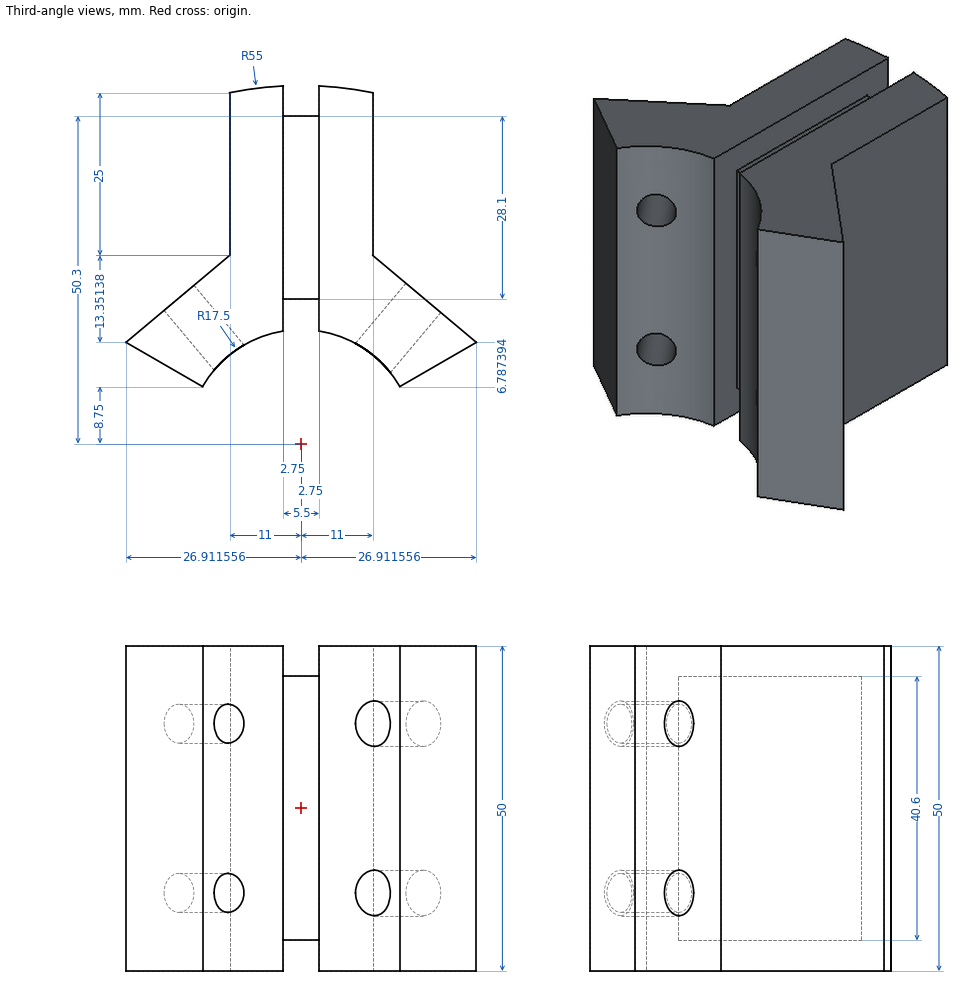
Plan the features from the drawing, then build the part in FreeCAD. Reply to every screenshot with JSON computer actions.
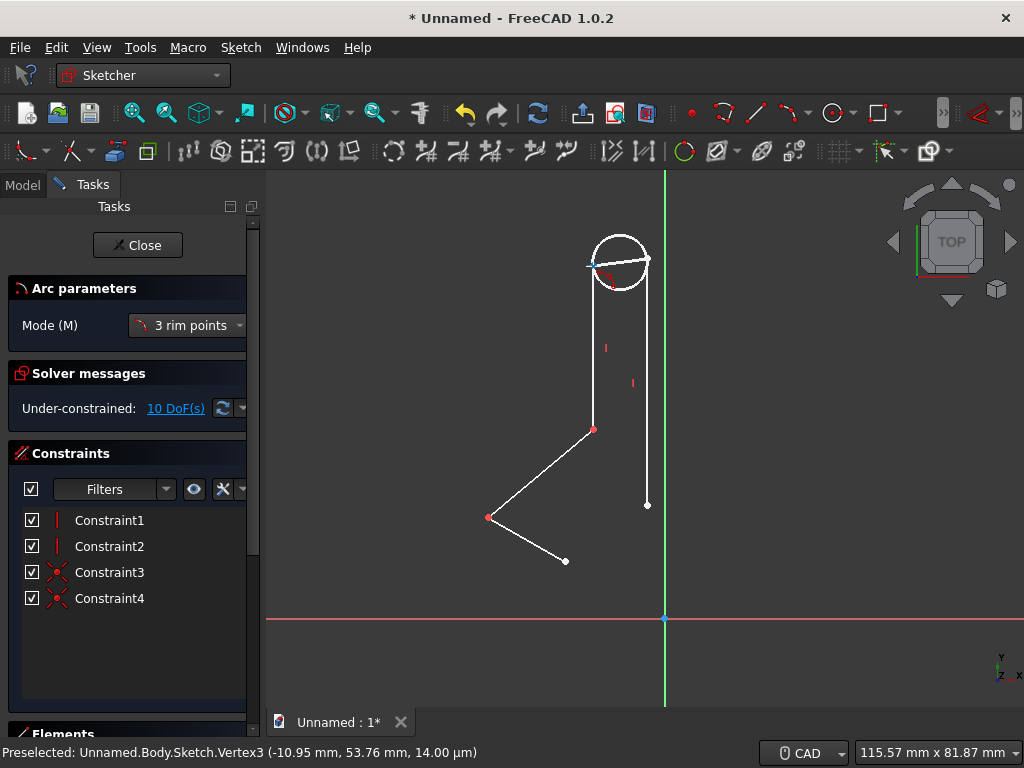
{"action": "scroll", "coordinate": [620, 261], "scroll_direction": "up", "scroll_amount": 14}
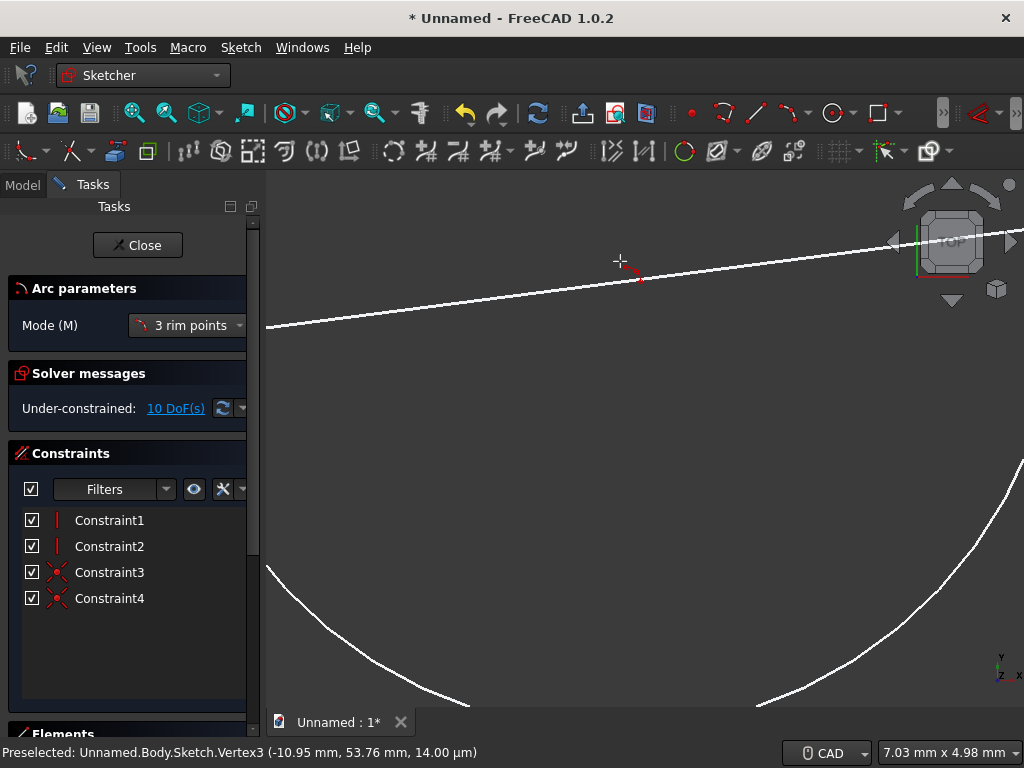
{"action": "left_click", "coordinate": [606, 254]}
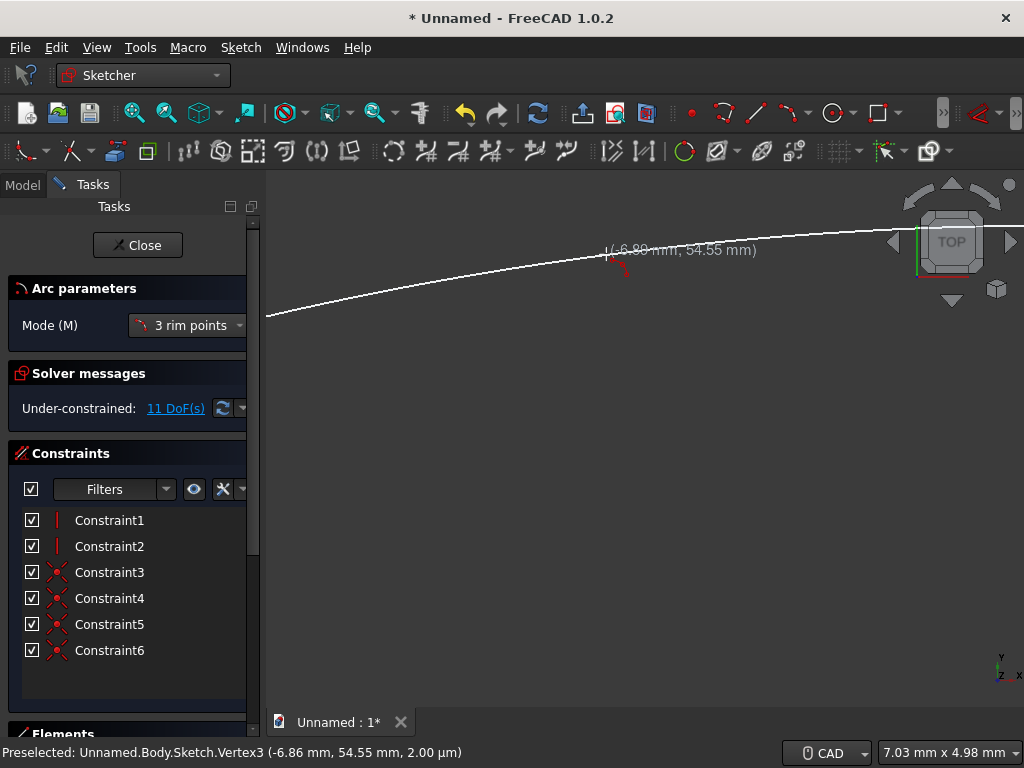
{"action": "scroll", "coordinate": [620, 261], "scroll_direction": "down", "scroll_amount": 14}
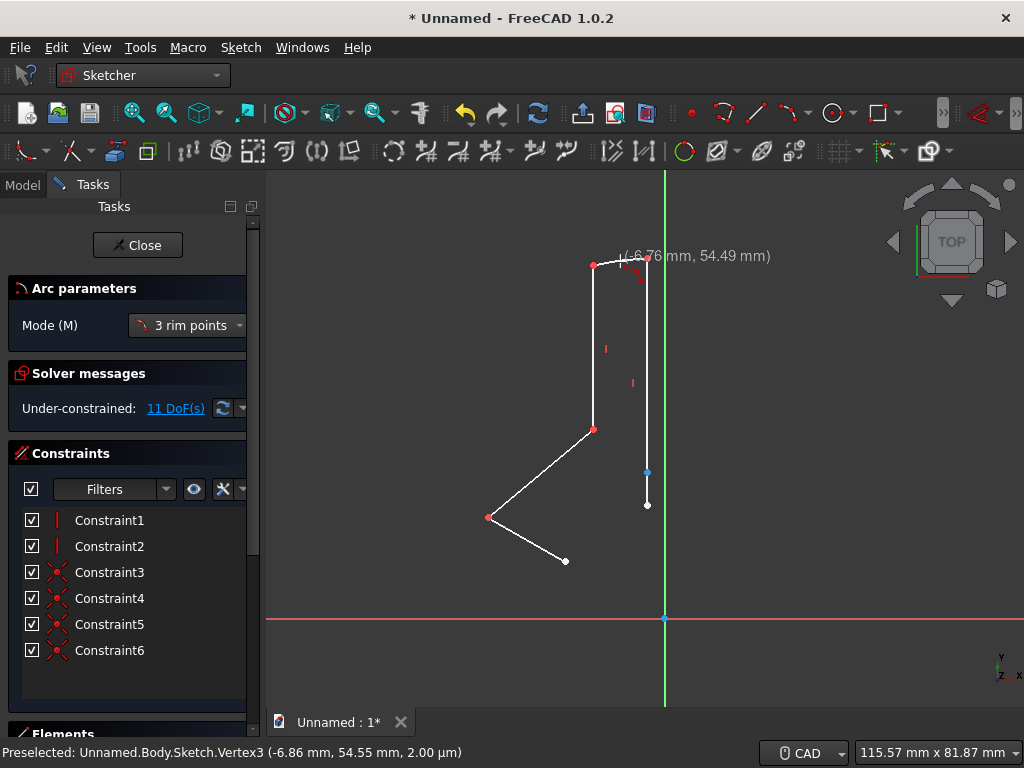
{"action": "left_click", "coordinate": [565, 562]}
{"action": "left_click", "coordinate": [647, 506]}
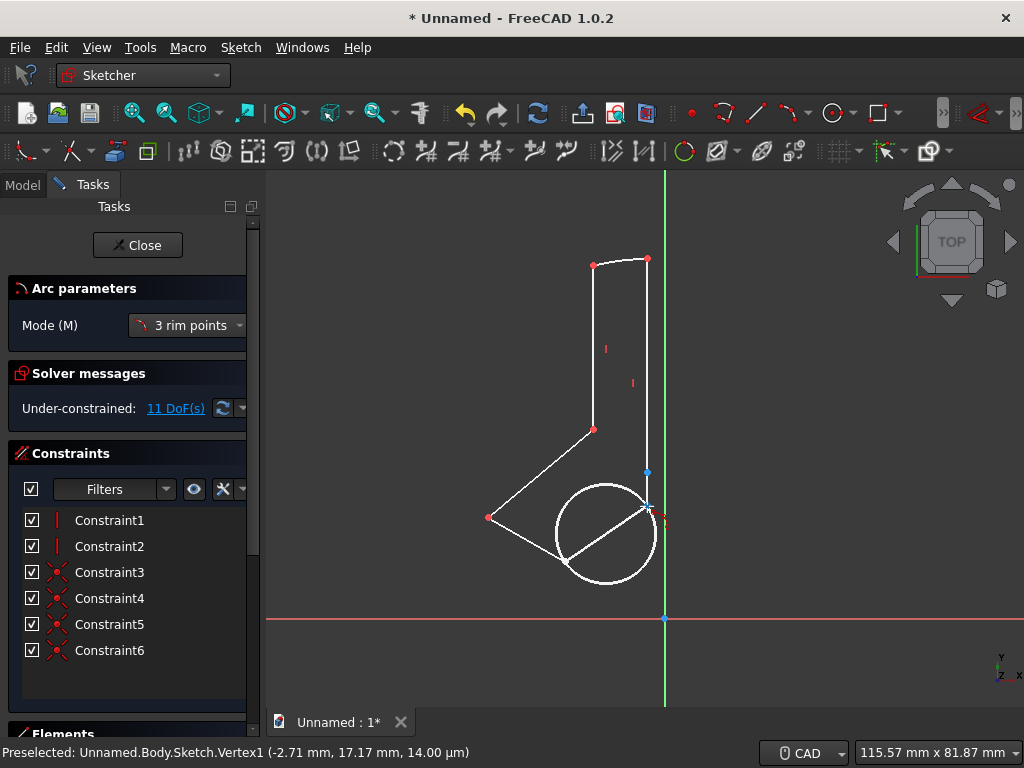
{"action": "scroll", "coordinate": [600, 524], "scroll_direction": "up", "scroll_amount": 2}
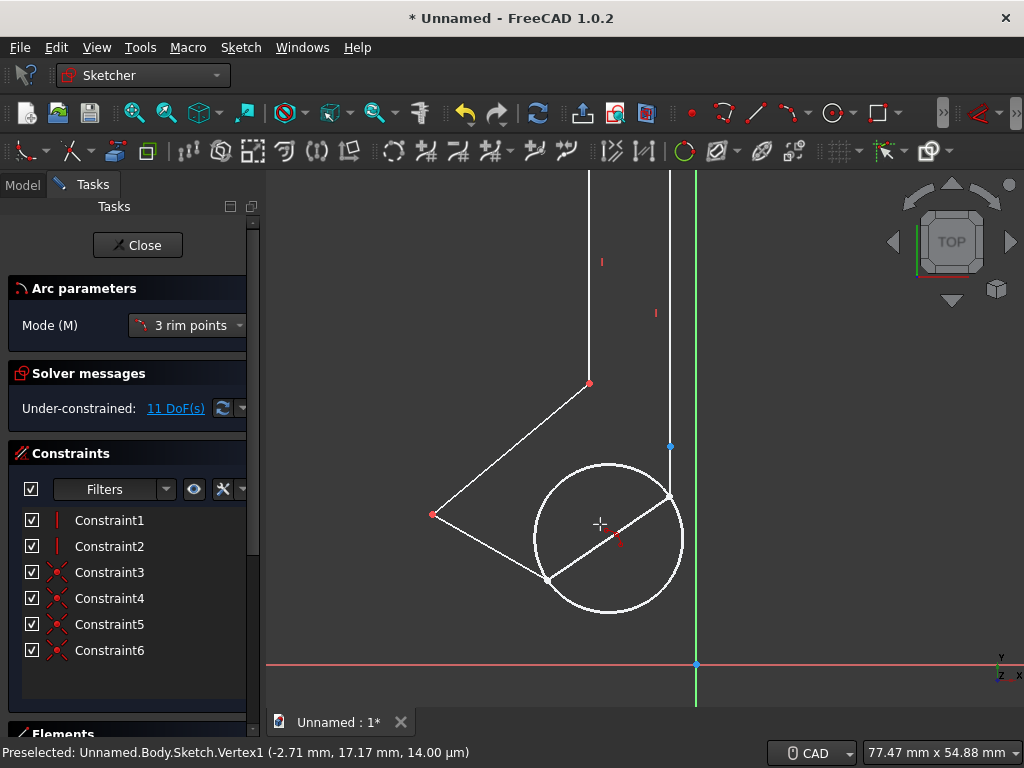
{"action": "left_click", "coordinate": [599, 524]}
{"action": "key", "text": "Escape"}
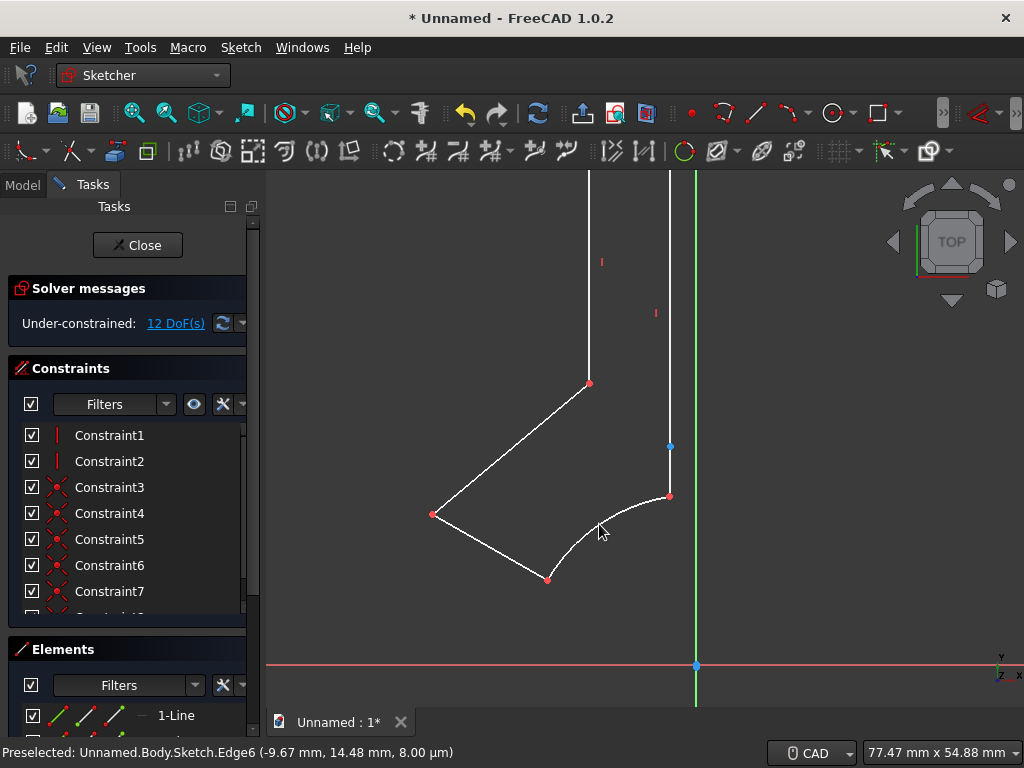
{"action": "scroll", "coordinate": [600, 525], "scroll_direction": "down", "scroll_amount": 2}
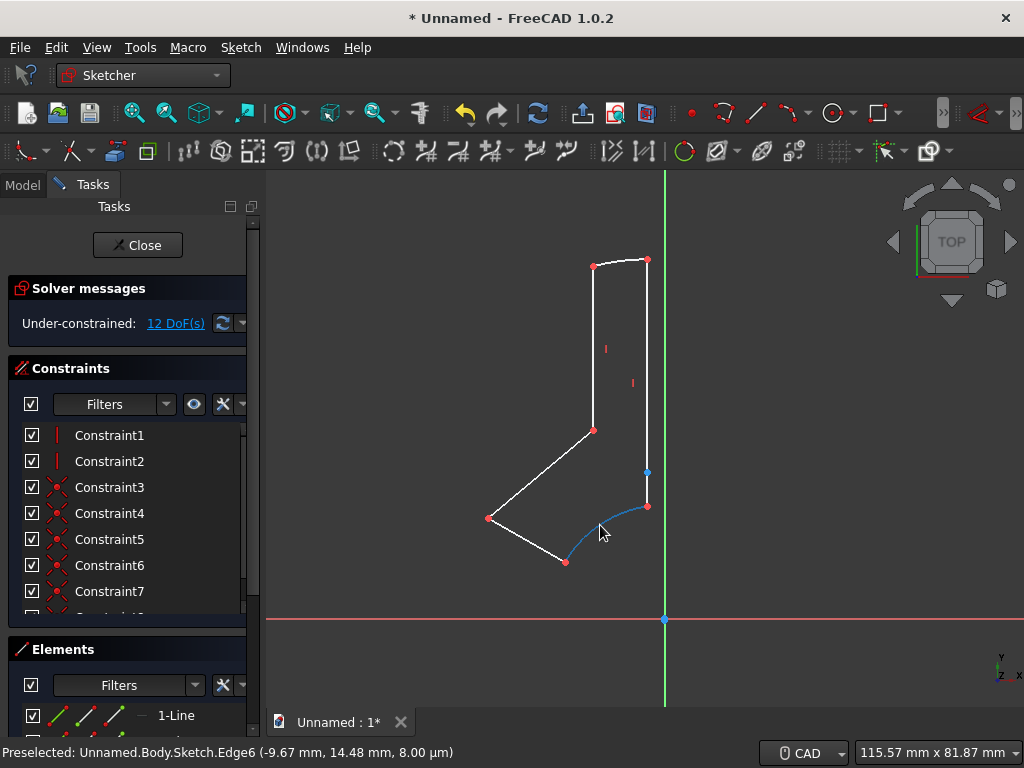
{"action": "left_click", "coordinate": [631, 260]}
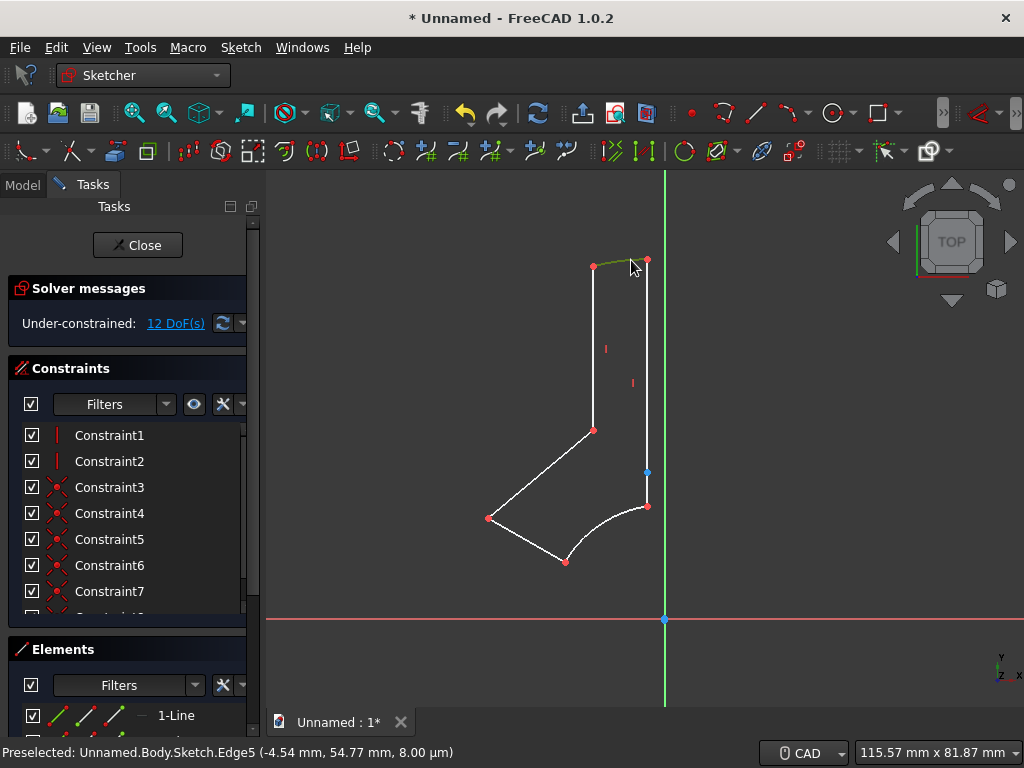
{"action": "left_click", "coordinate": [618, 515]}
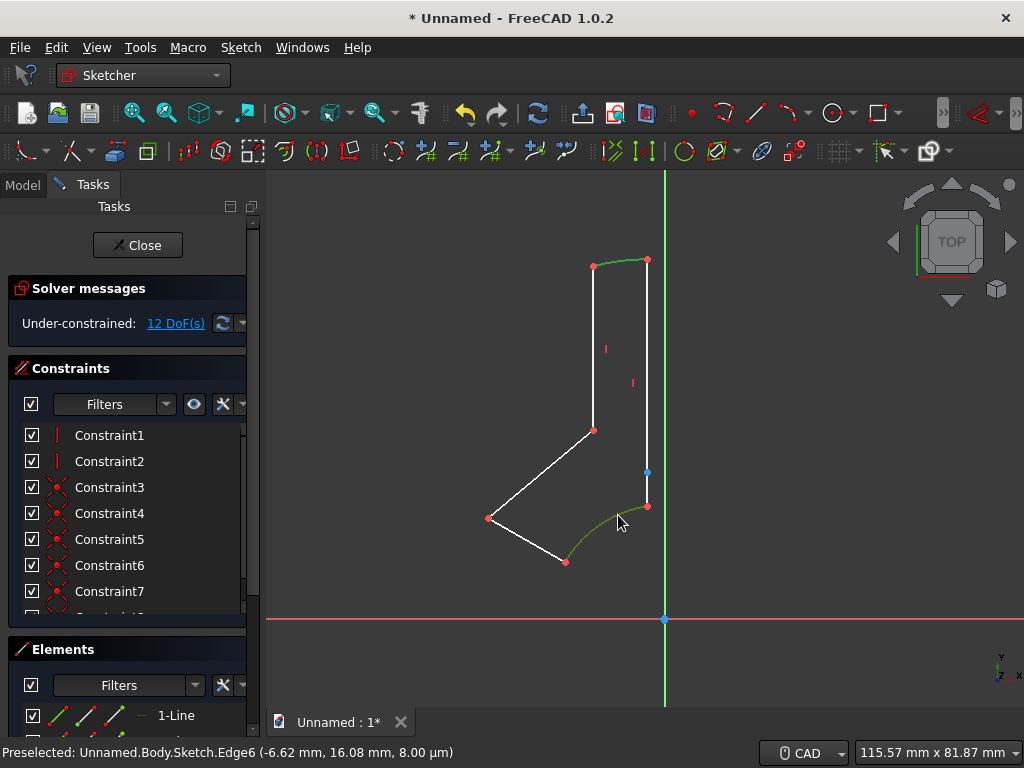
{"action": "key", "text": "c"}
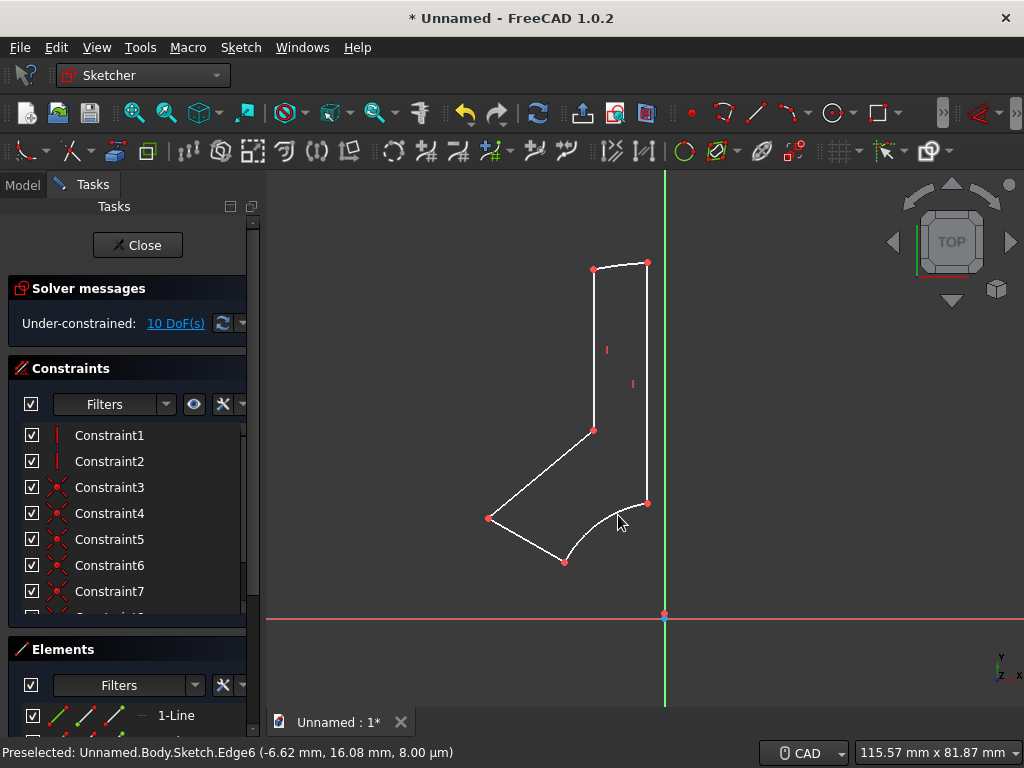
{"action": "left_click_drag", "start_coordinate": [654, 604], "coordinate": [675, 629]}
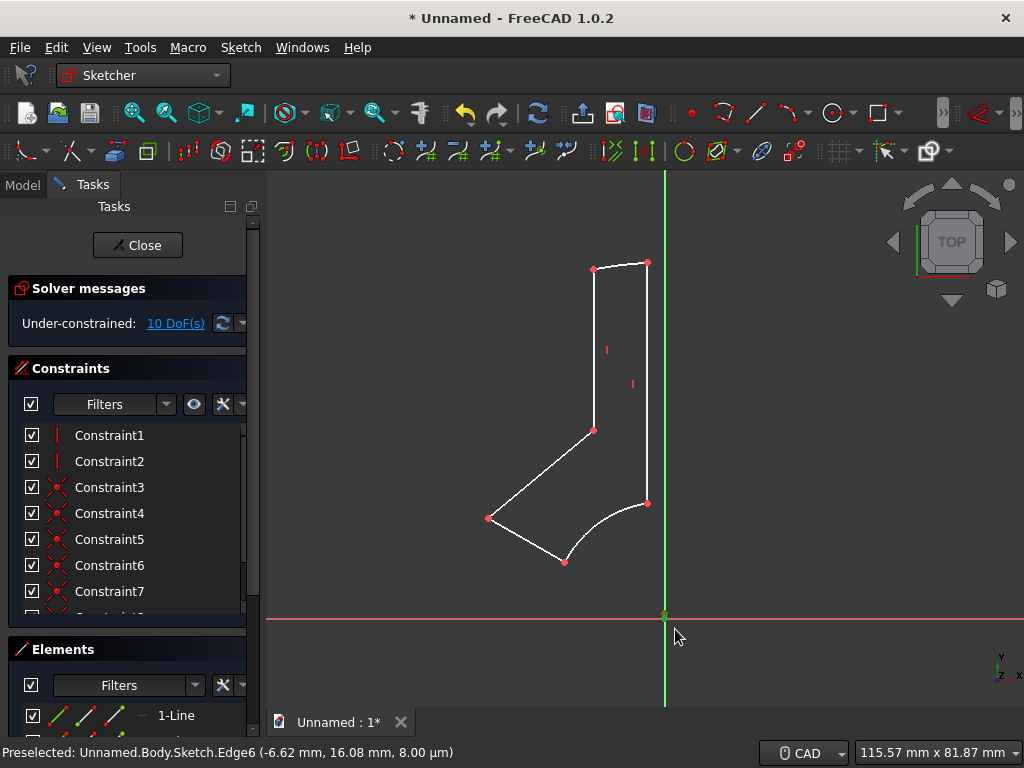
{"action": "key", "text": "c"}